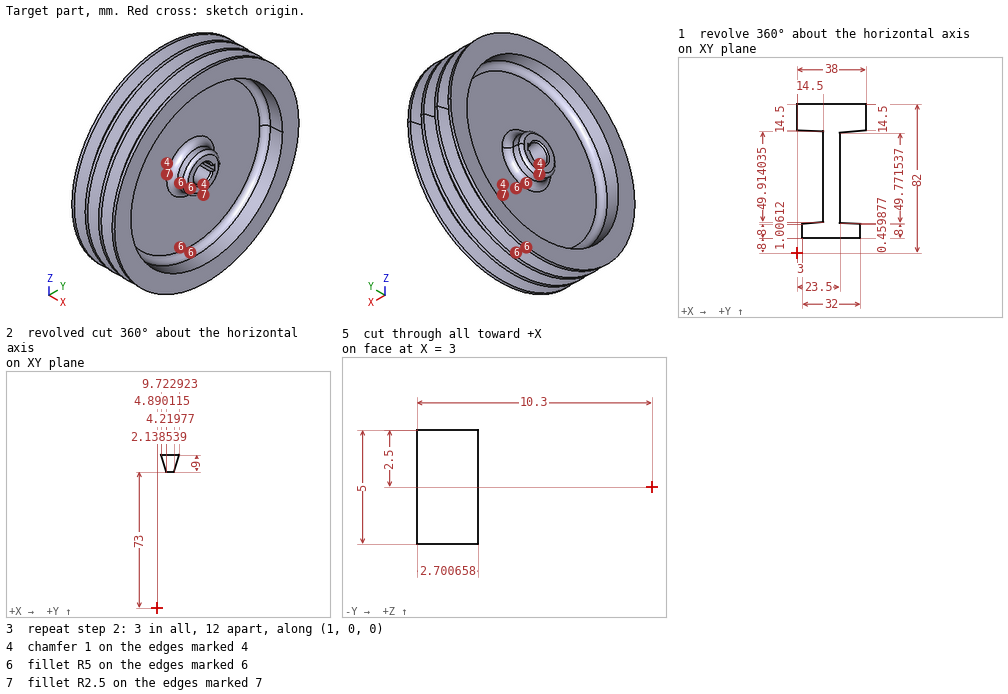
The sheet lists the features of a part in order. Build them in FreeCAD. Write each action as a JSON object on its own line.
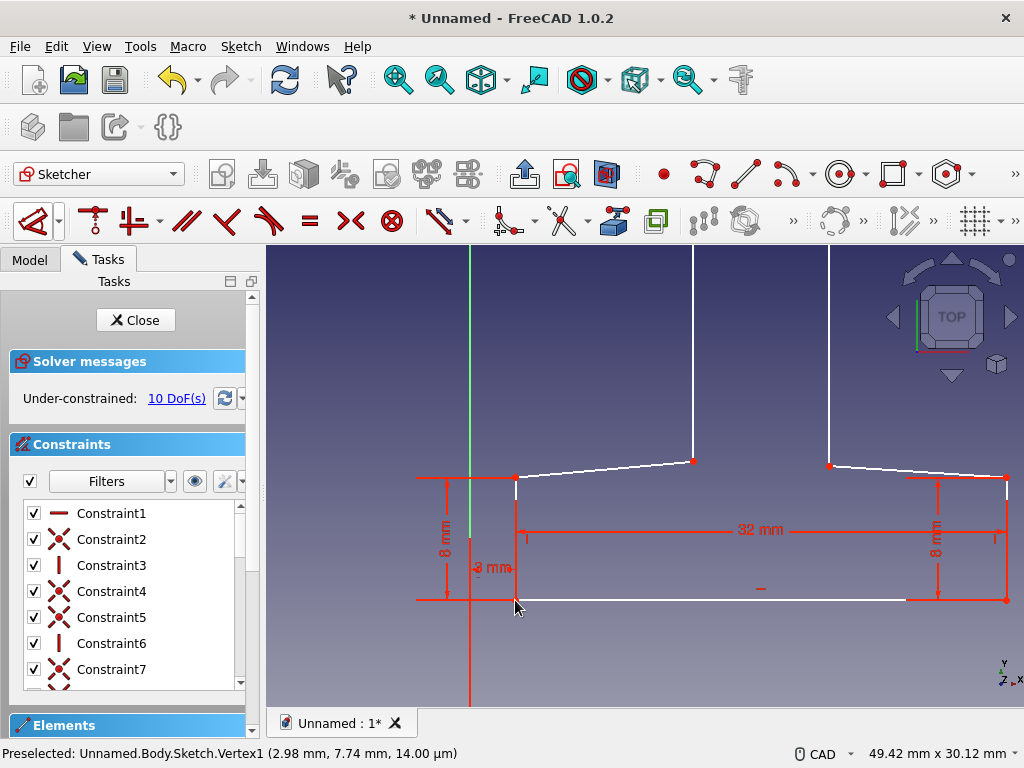
{"action": "scroll", "coordinate": [516, 602], "scroll_direction": "down", "scroll_amount": 7}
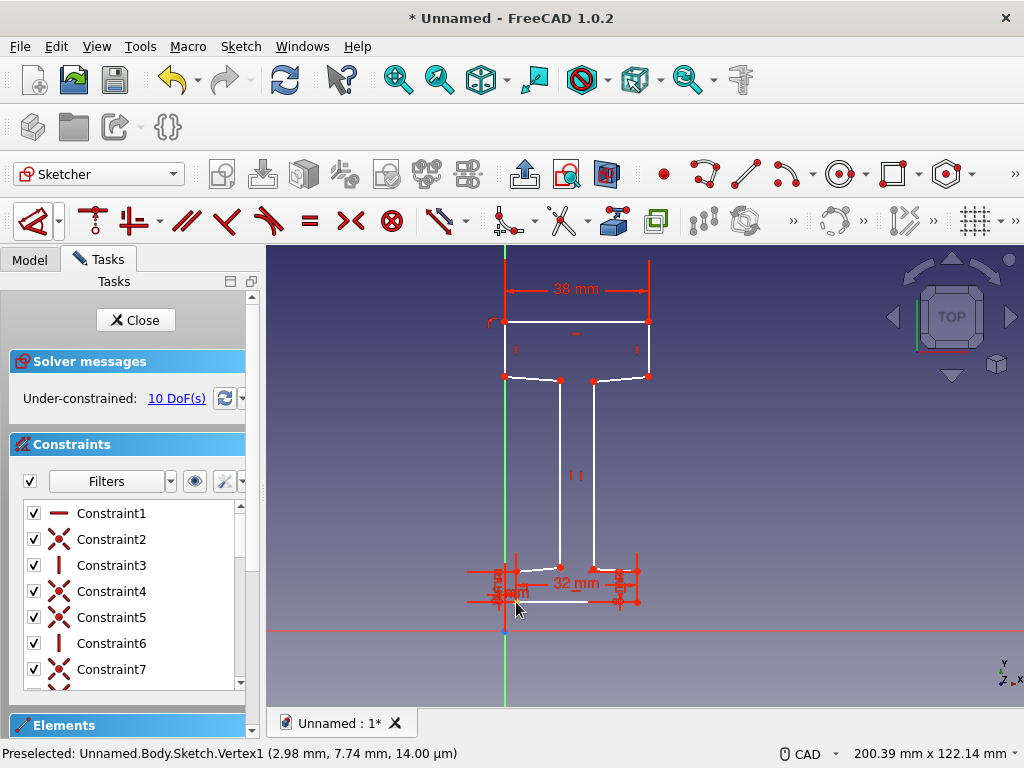
{"action": "scroll", "coordinate": [516, 602], "scroll_direction": "up", "scroll_amount": 2}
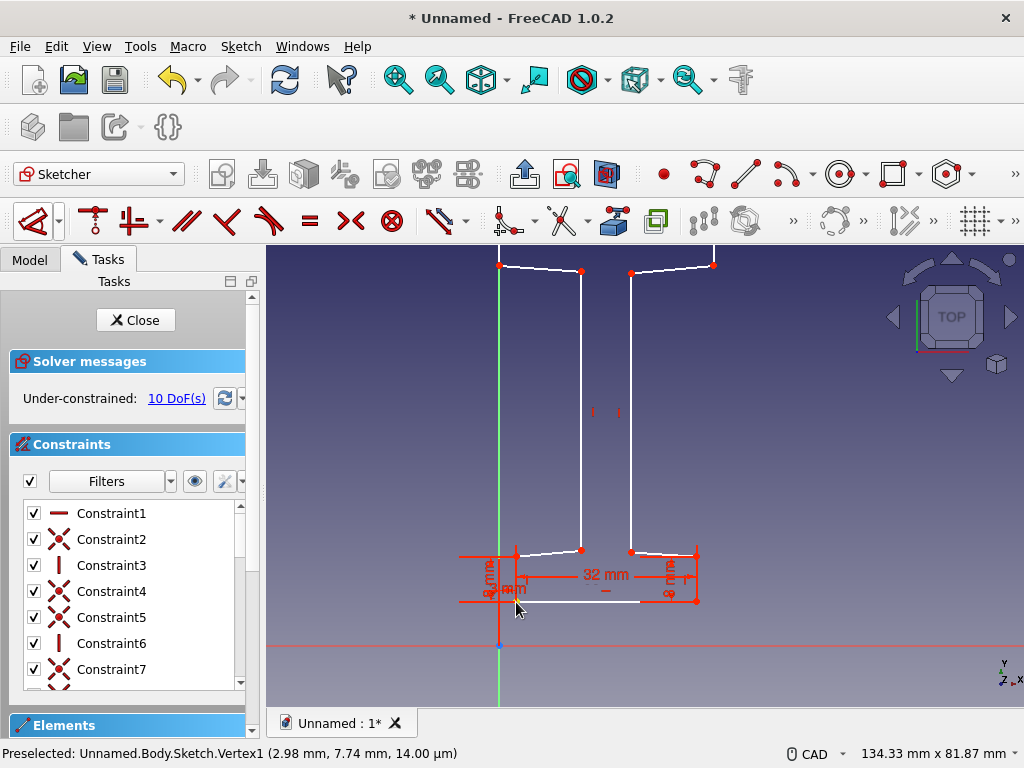
{"action": "left_click", "coordinate": [516, 602]}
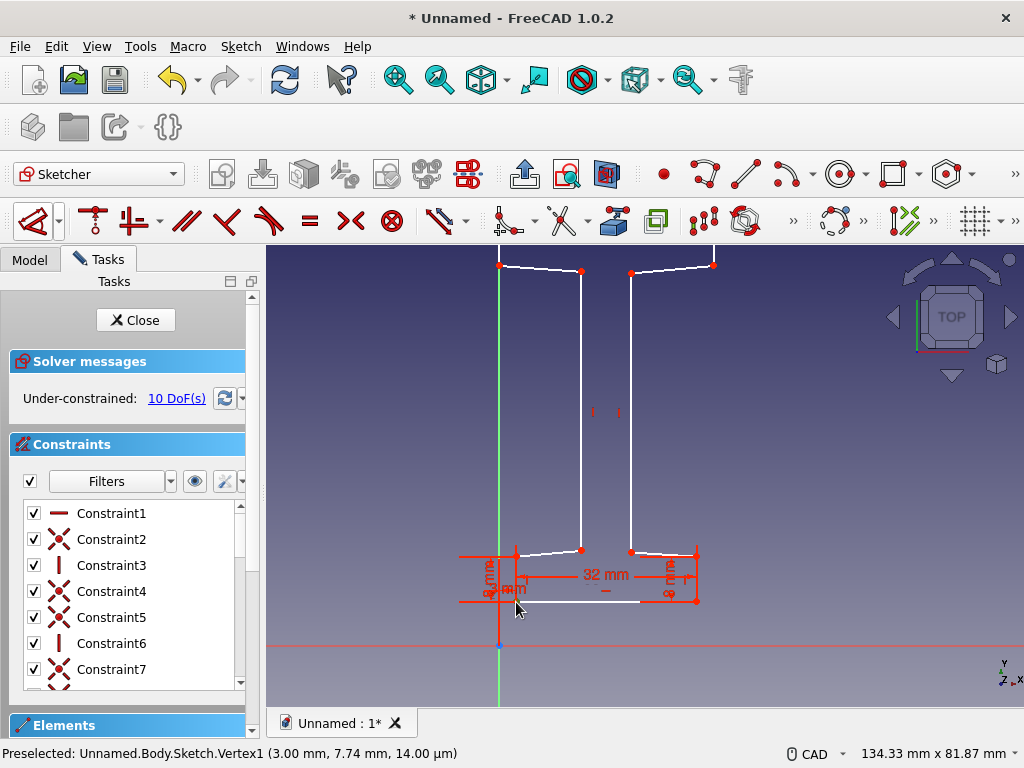
{"action": "left_click", "coordinate": [58, 222]}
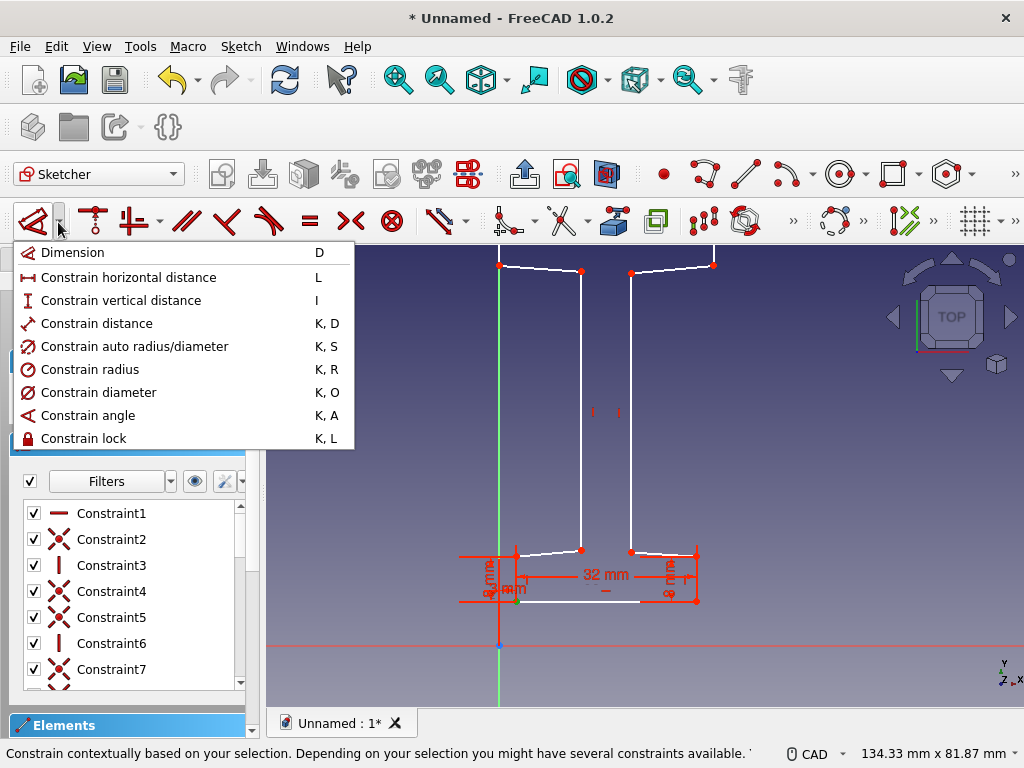
{"action": "left_click", "coordinate": [184, 300]}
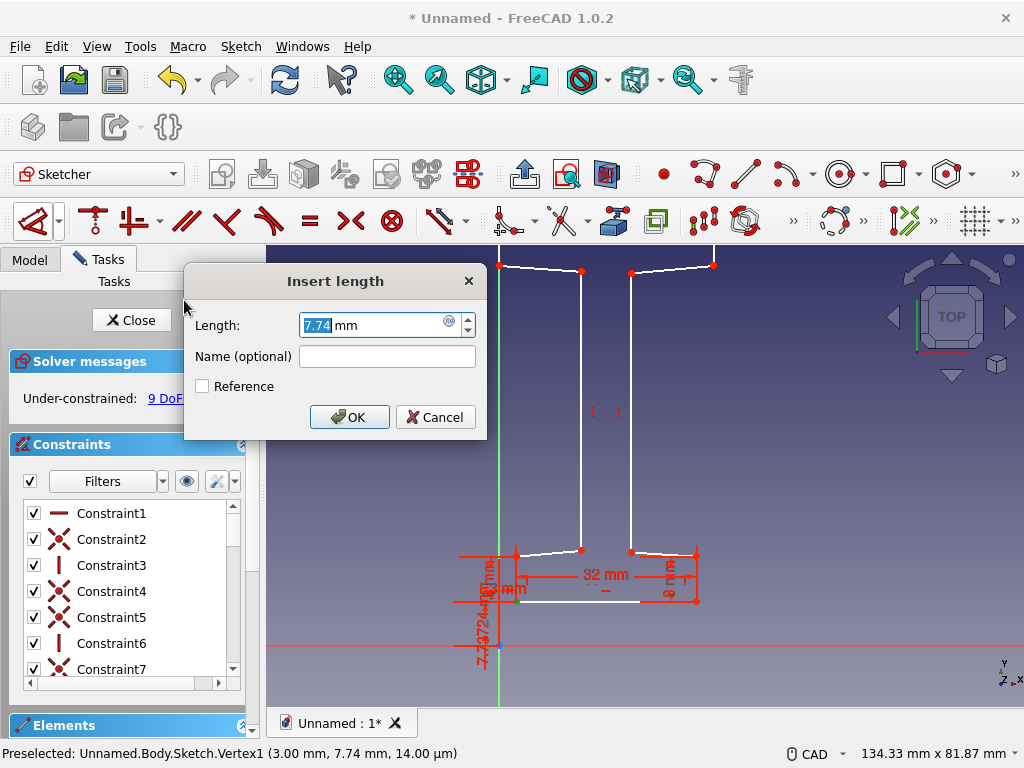
{"action": "type", "text": "8"}
{"action": "key", "text": "Return"}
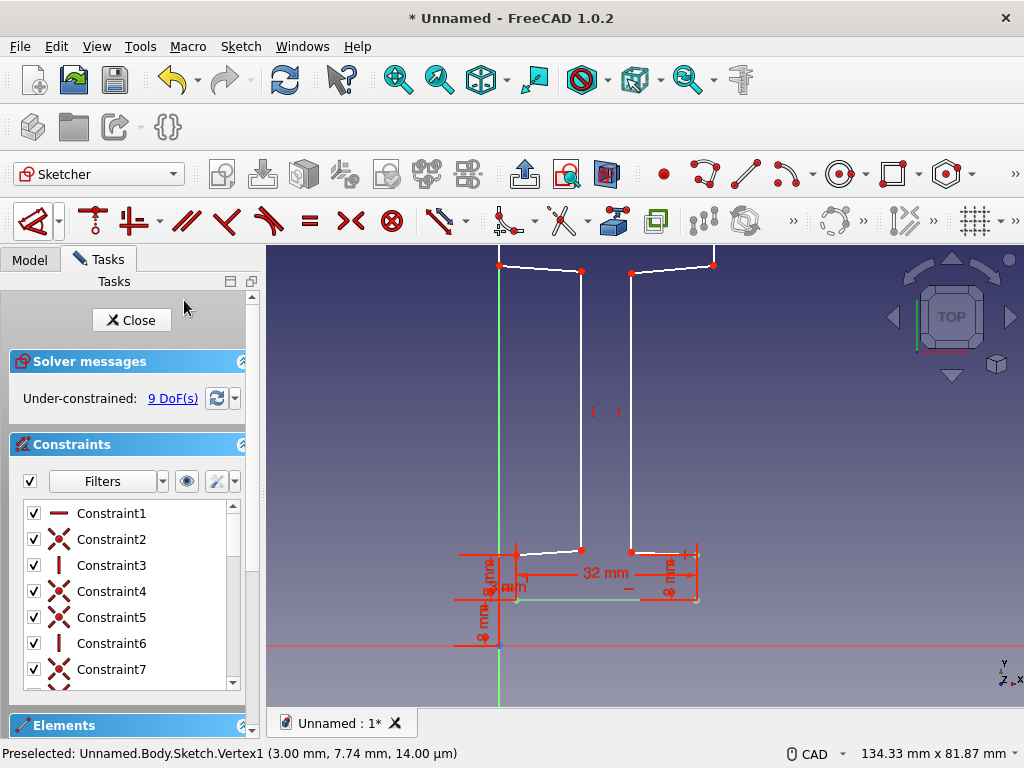
{"action": "scroll", "coordinate": [516, 602], "scroll_direction": "down", "scroll_amount": 2}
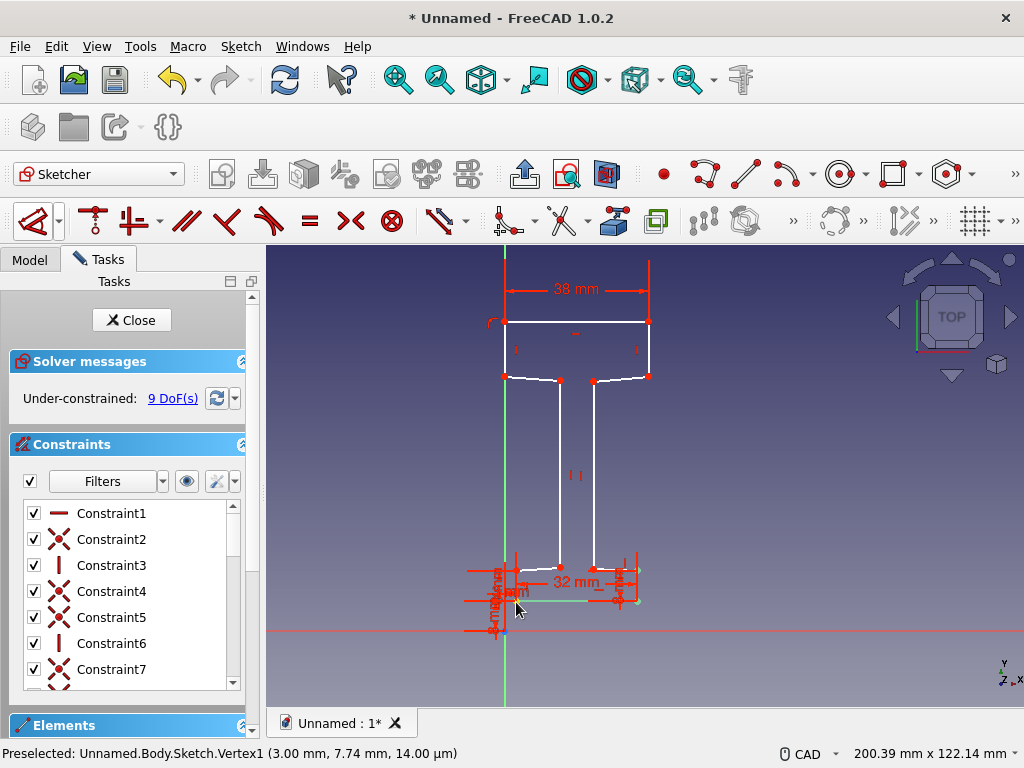
{"action": "left_click", "coordinate": [649, 322]}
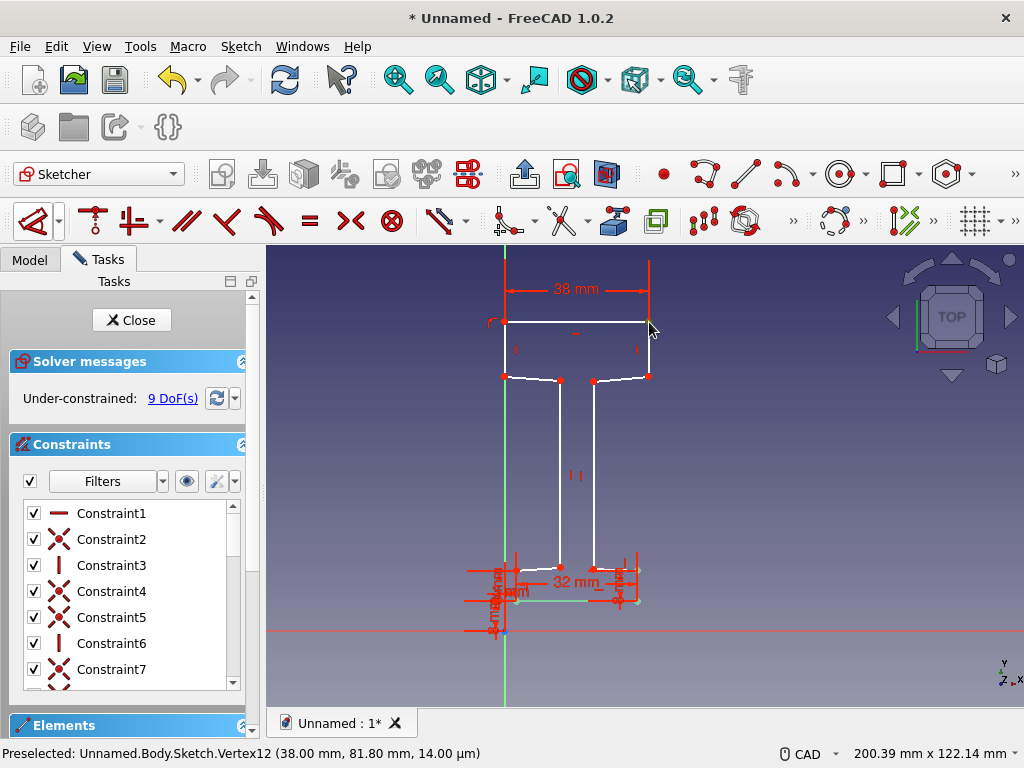
{"action": "key", "text": "i"}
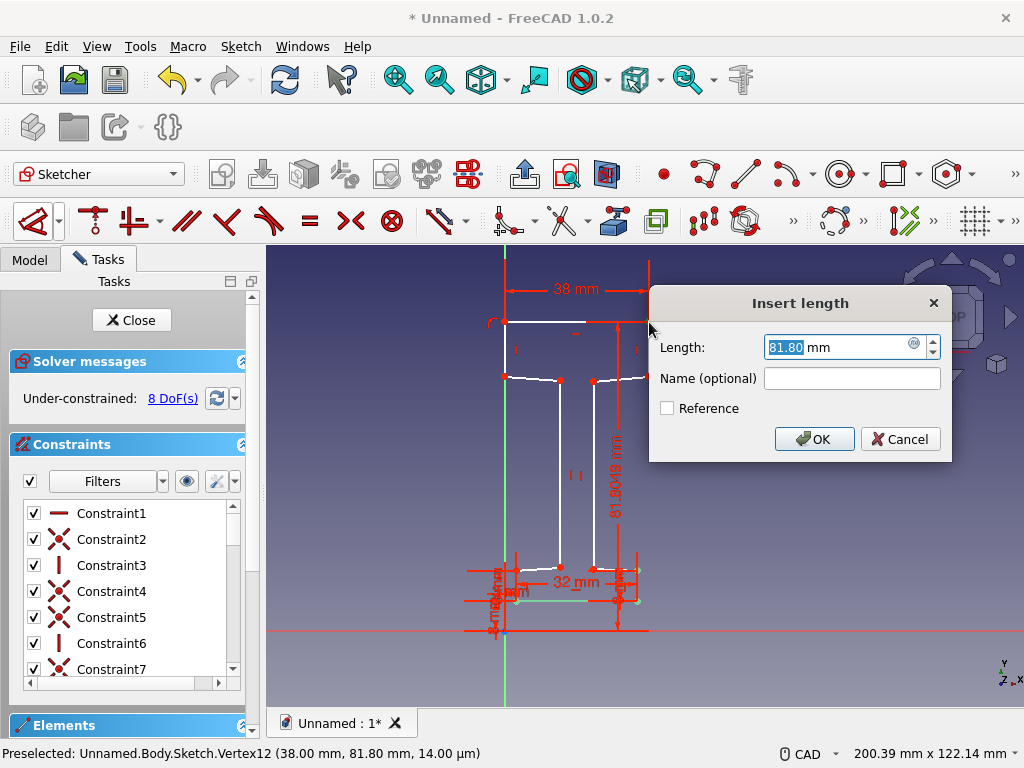
{"action": "type", "text": "82"}
{"action": "key", "text": "Return"}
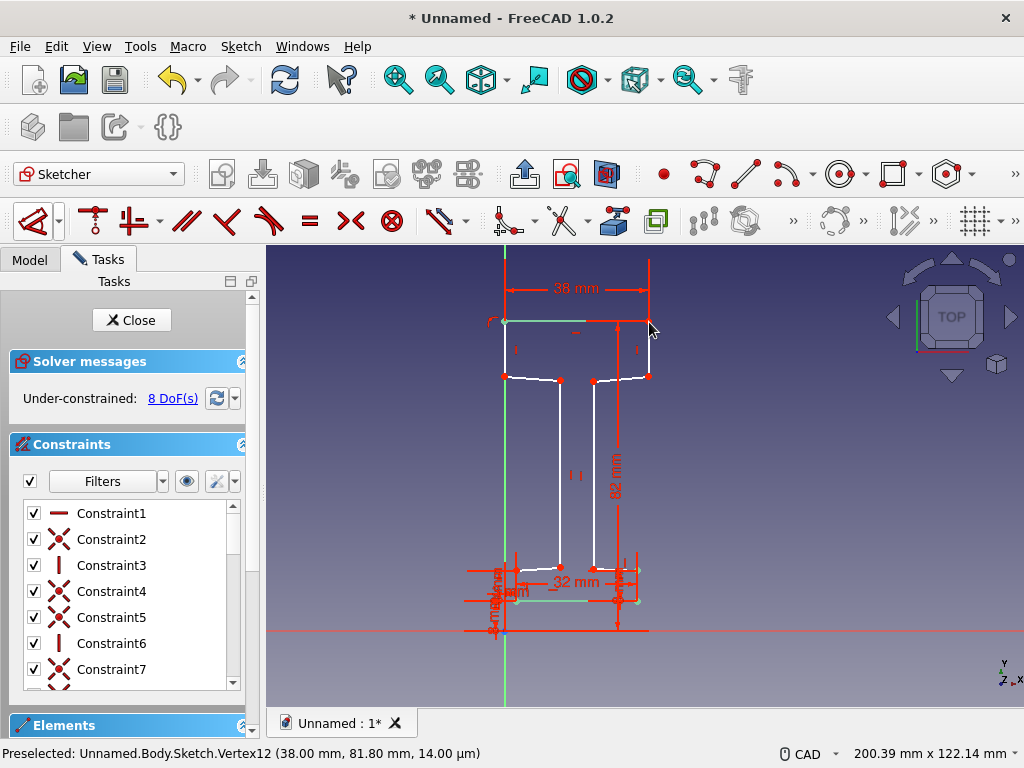
{"action": "left_click", "coordinate": [649, 360]}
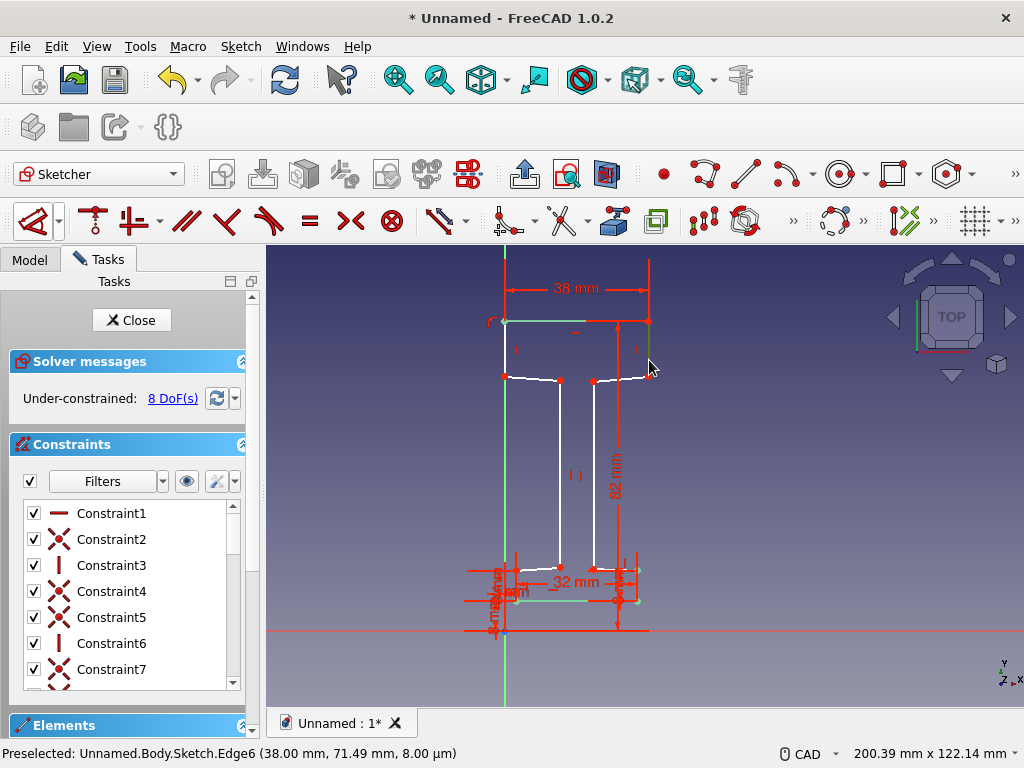
{"action": "left_click", "coordinate": [58, 222]}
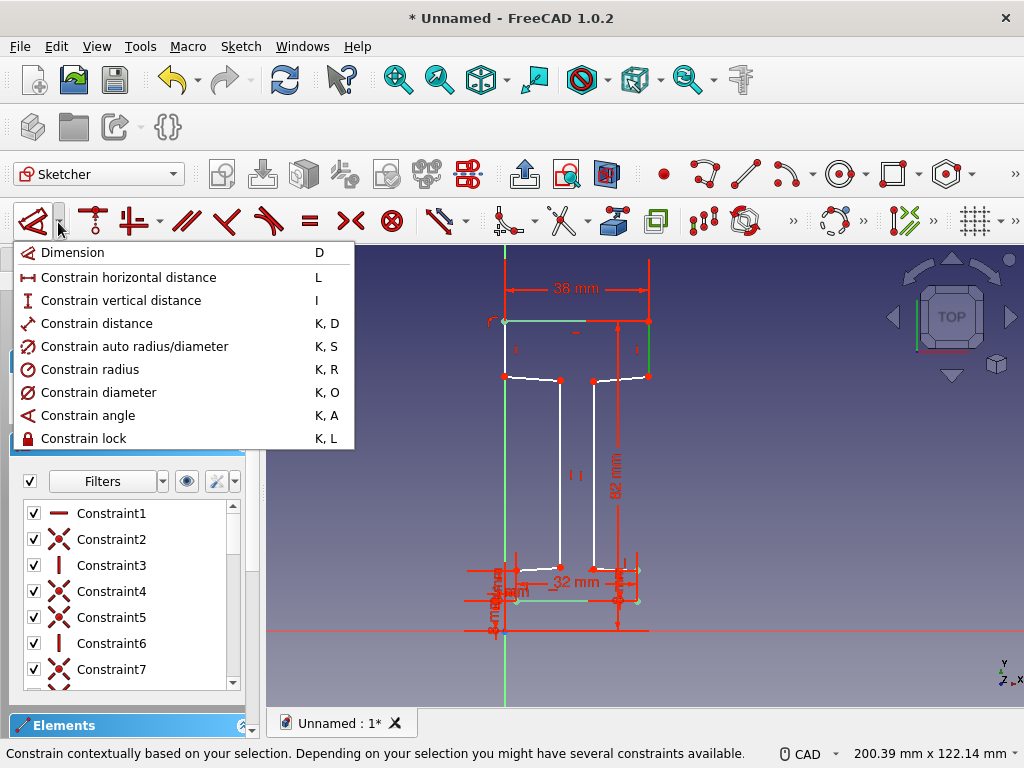
{"action": "left_click", "coordinate": [184, 300]}